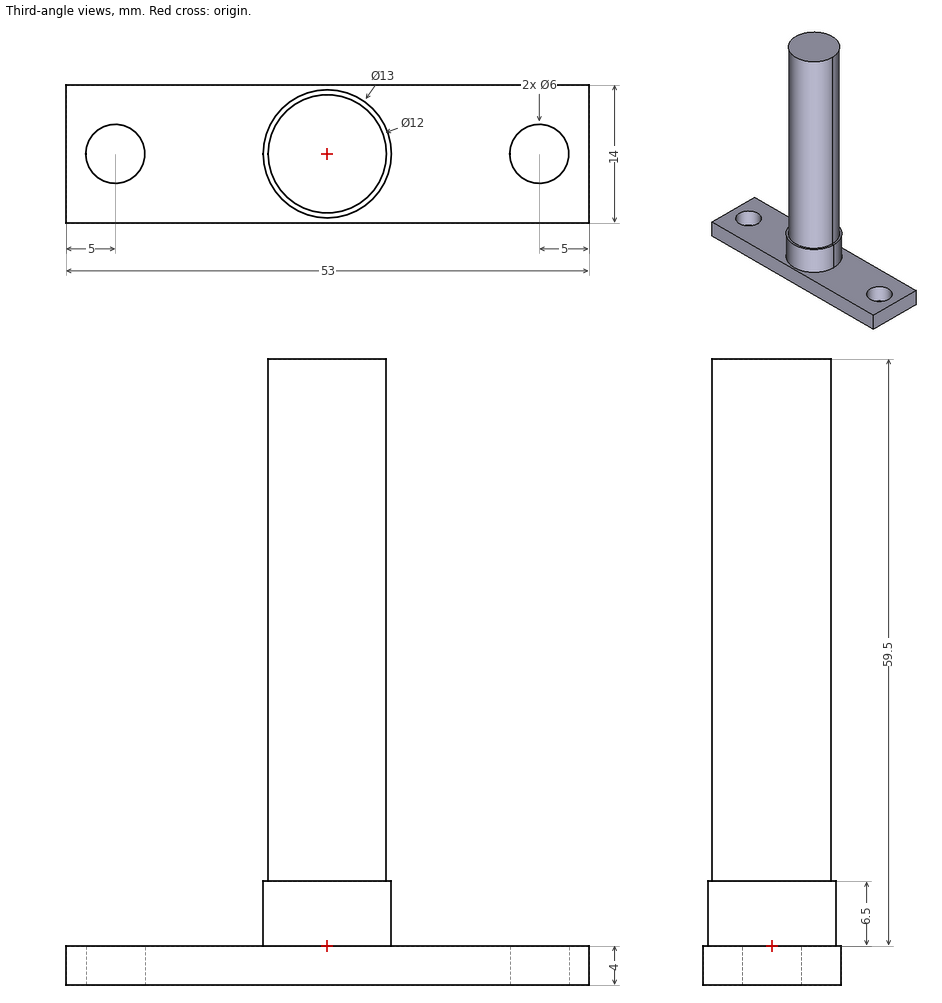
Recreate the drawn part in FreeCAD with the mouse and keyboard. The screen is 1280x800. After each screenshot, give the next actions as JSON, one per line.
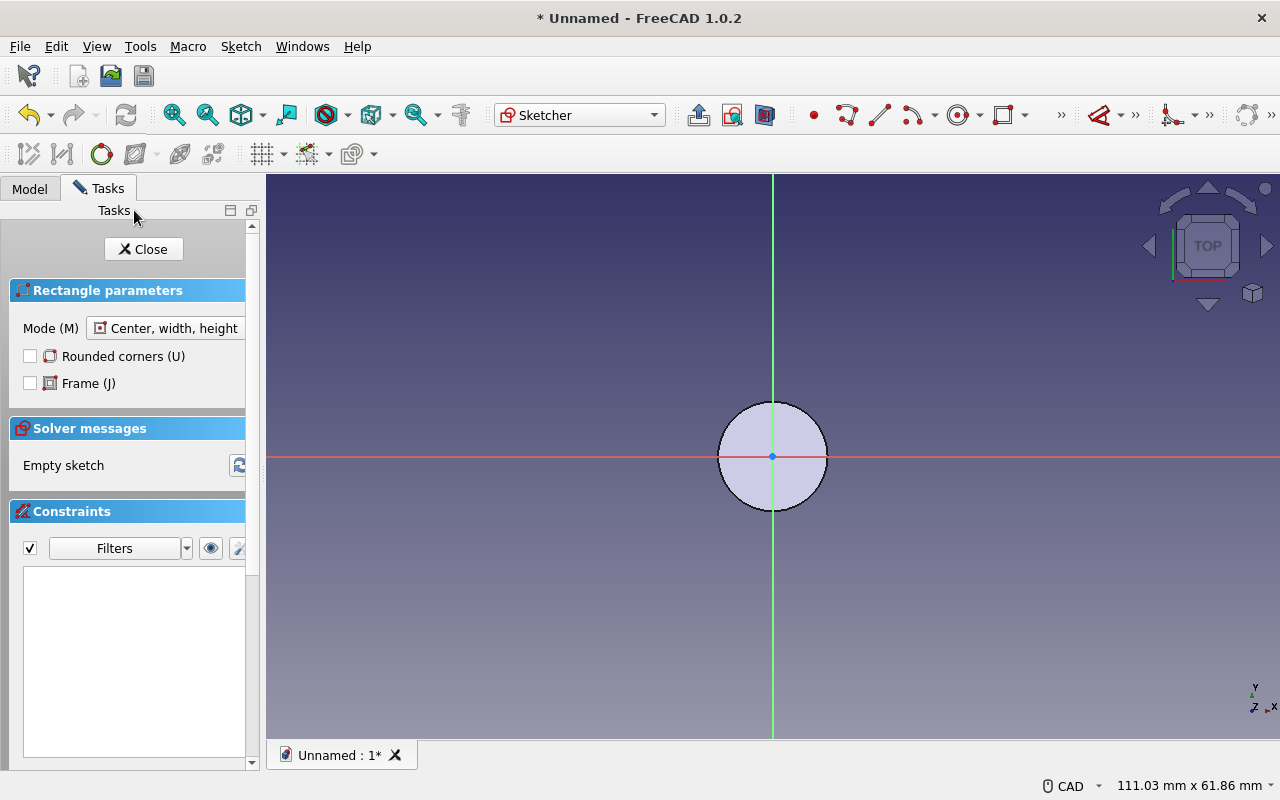
{"action": "left_click", "coordinate": [773, 456]}
{"action": "left_click", "coordinate": [1015, 393]}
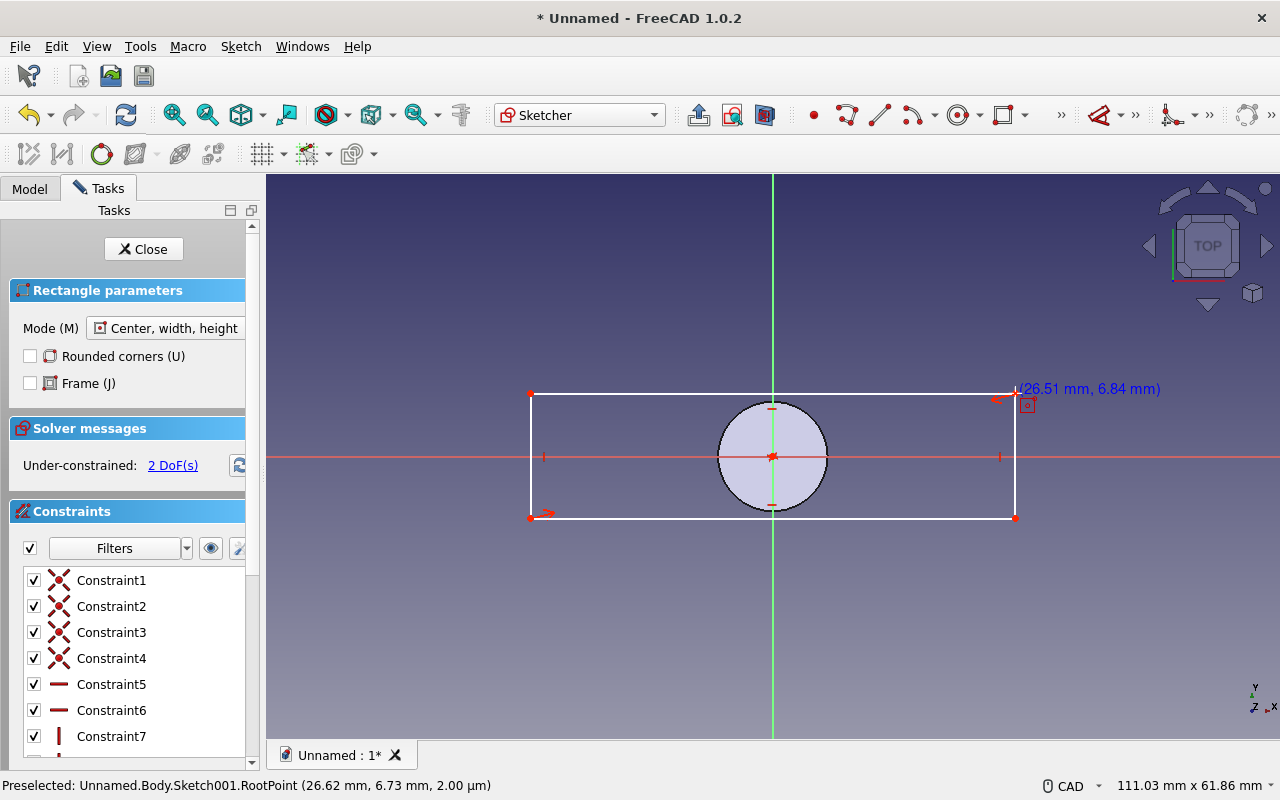
{"action": "key", "text": "g c"}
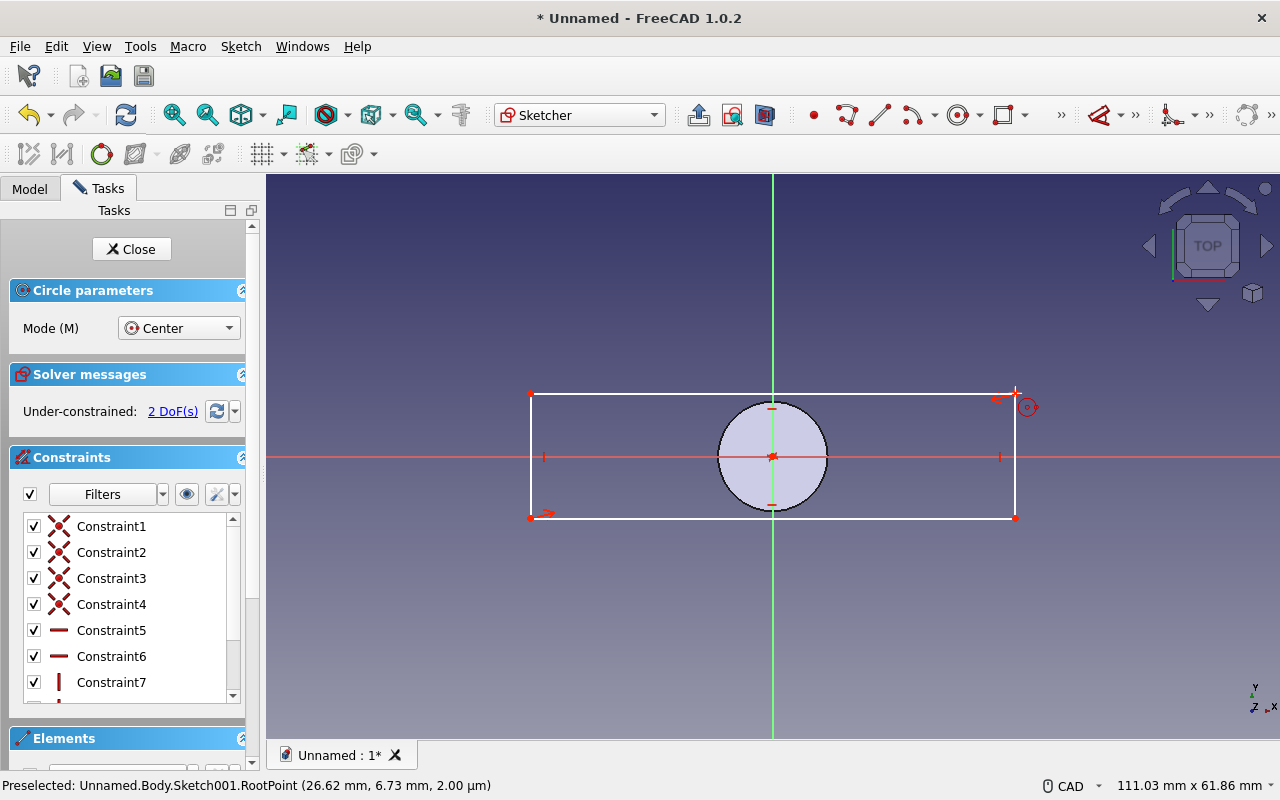
{"action": "left_click", "coordinate": [969, 456]}
{"action": "left_click", "coordinate": [989, 437]}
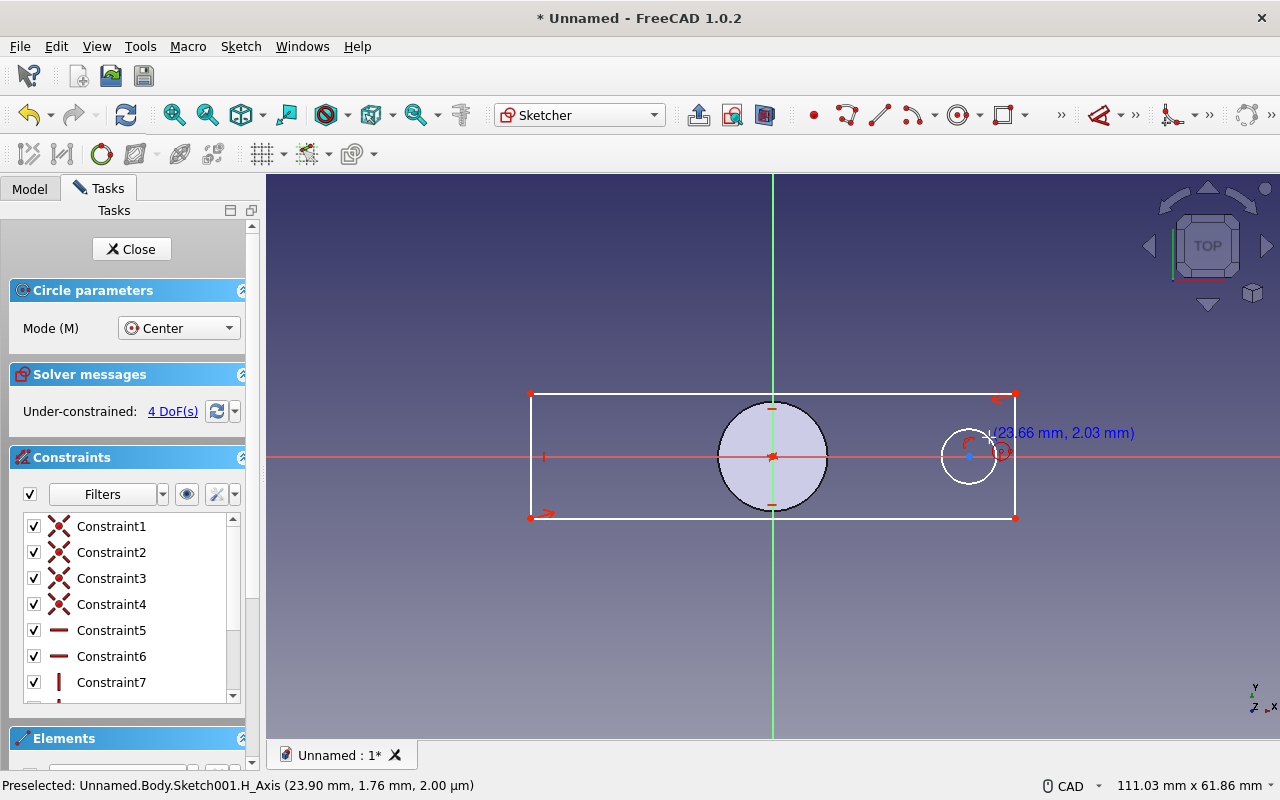
{"action": "left_click", "coordinate": [577, 456]}
{"action": "left_click", "coordinate": [596, 437]}
{"action": "key", "text": "Escape"}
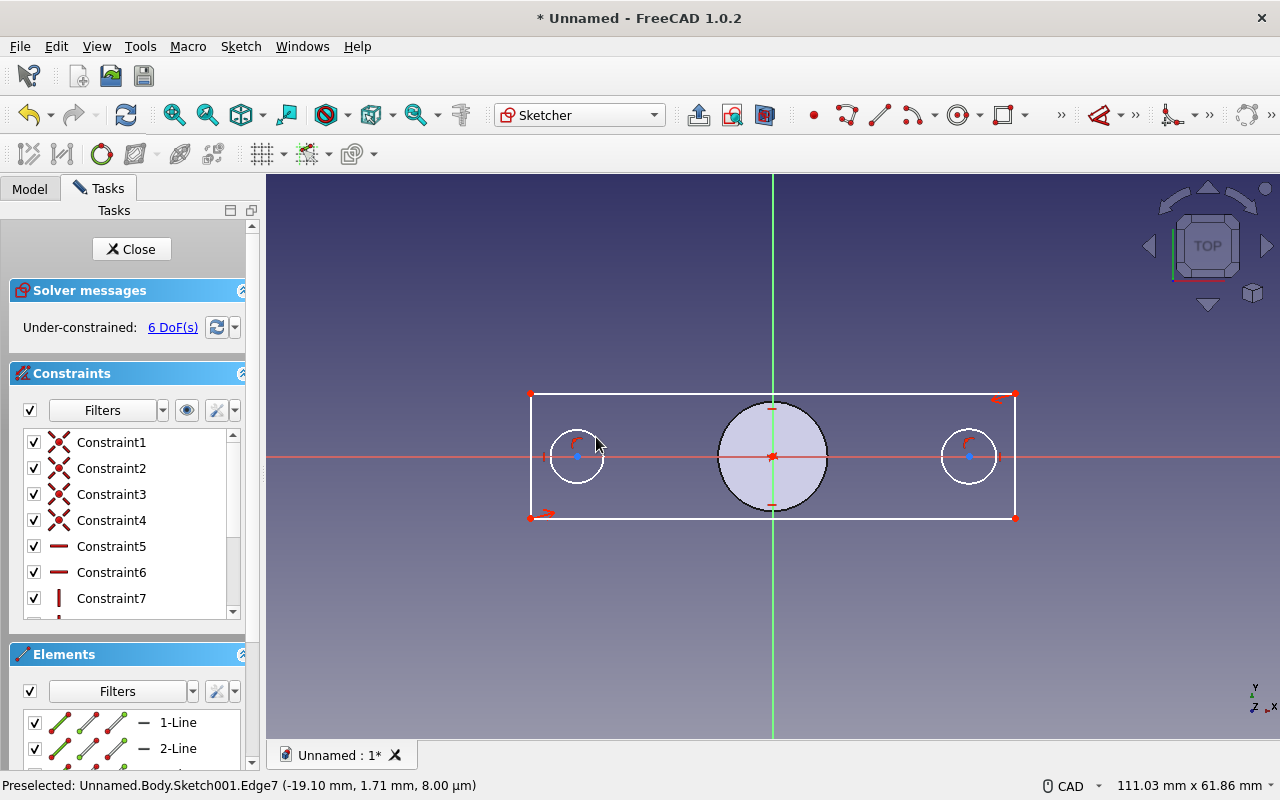
{"action": "left_click", "coordinate": [988, 437]}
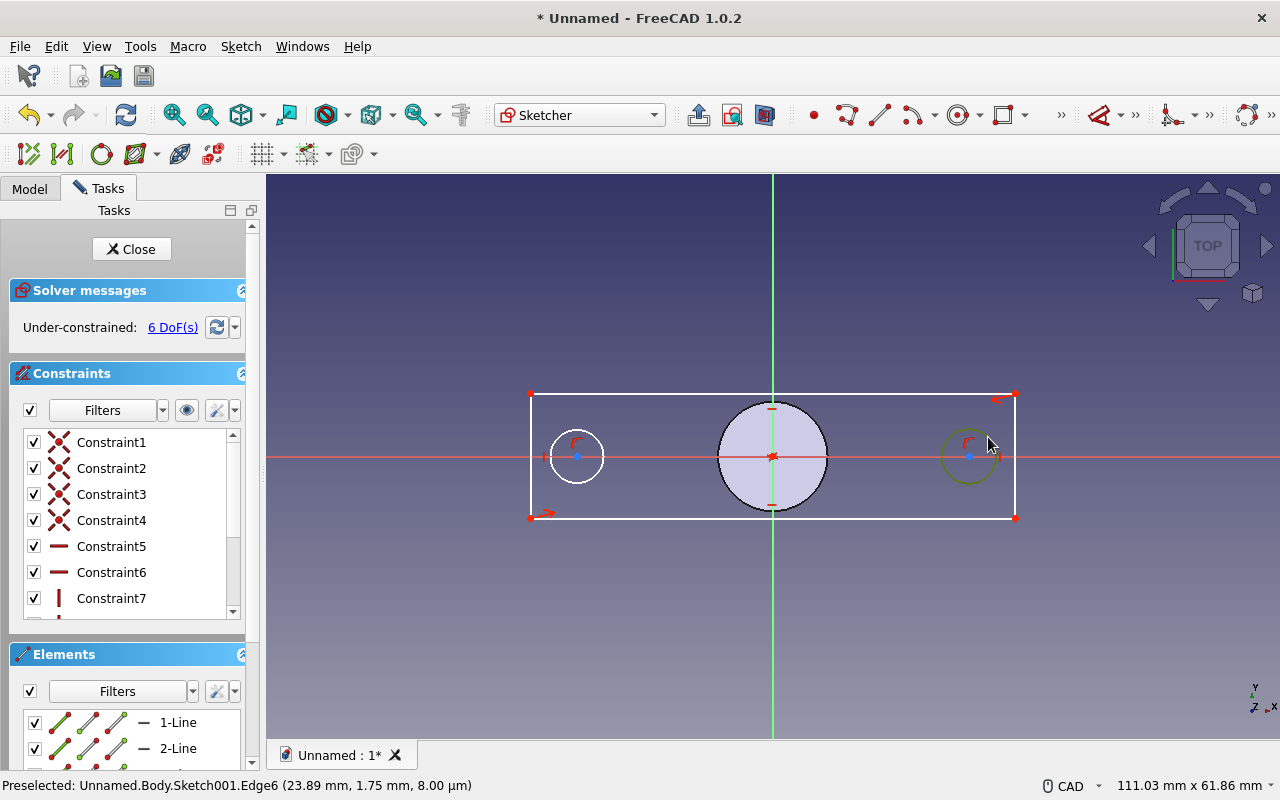
{"action": "left_click", "coordinate": [596, 438]}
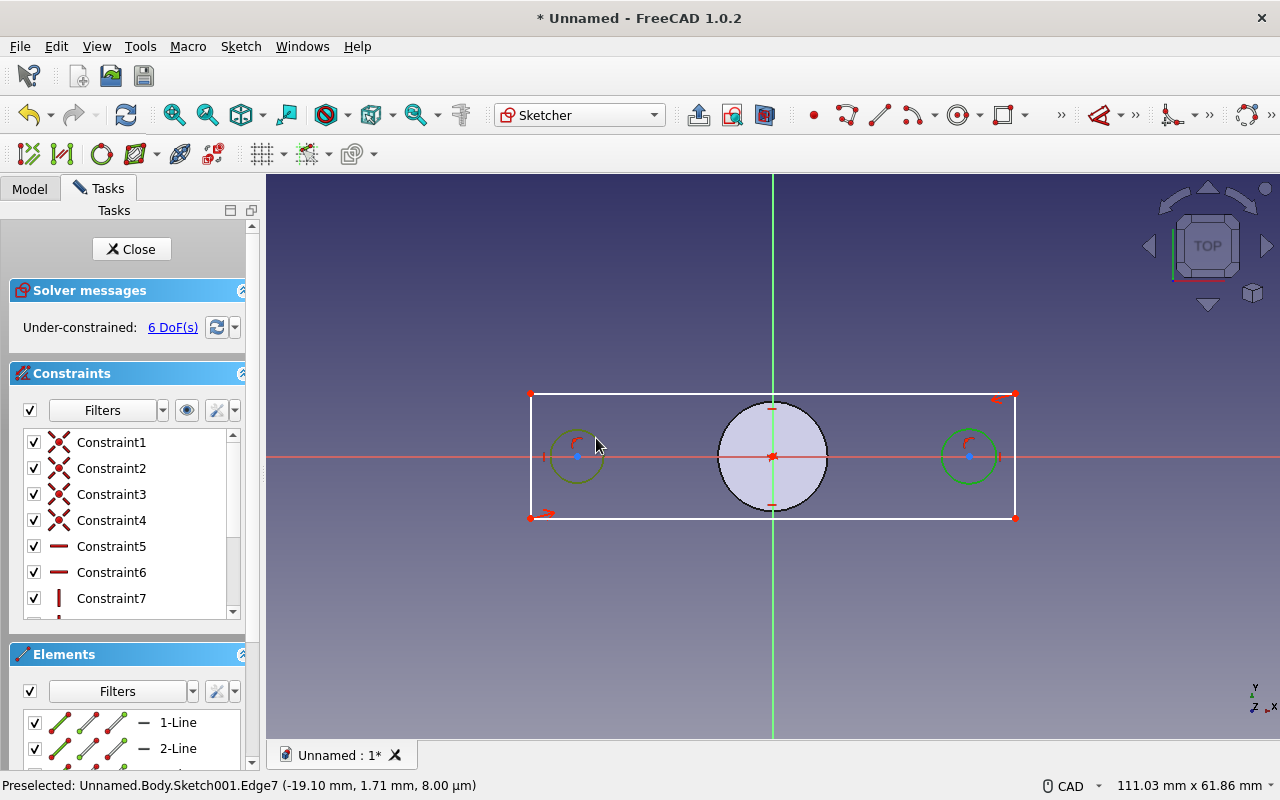
{"action": "key", "text": "e"}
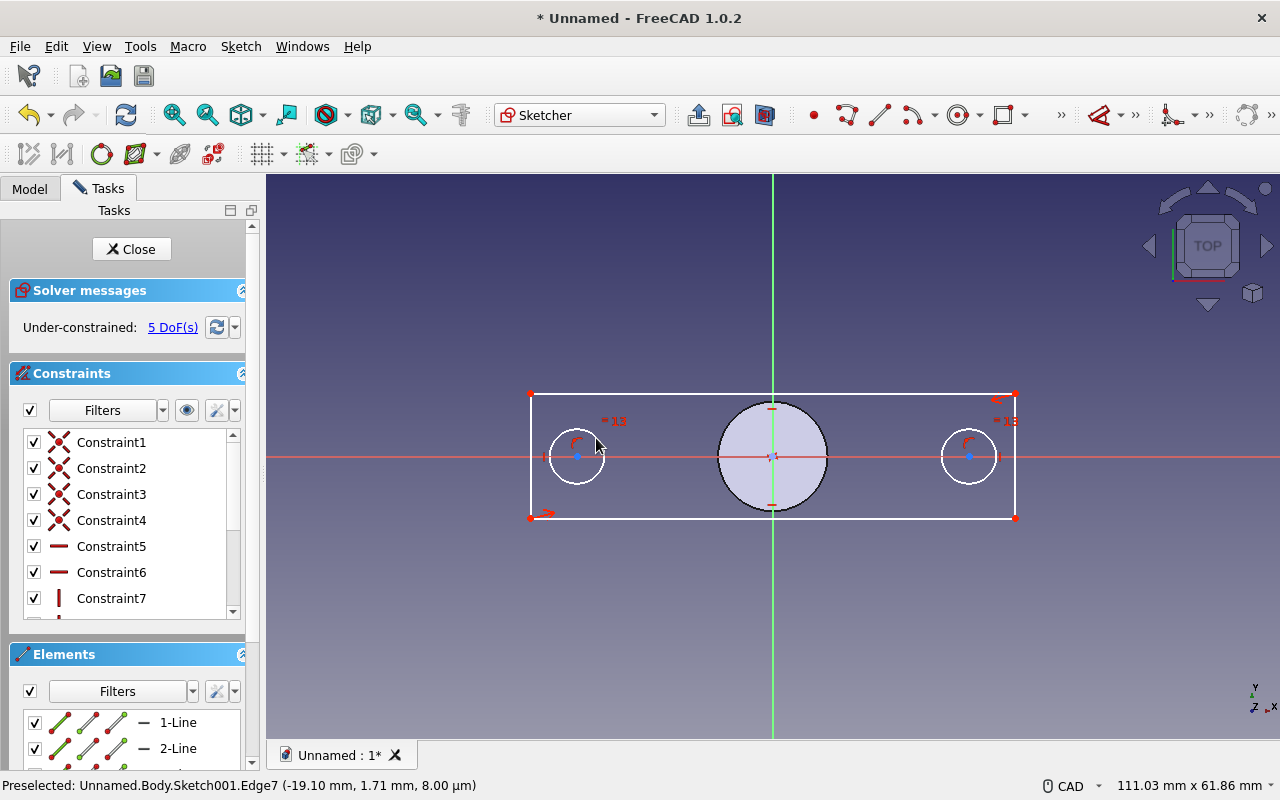
{"action": "key", "text": "d"}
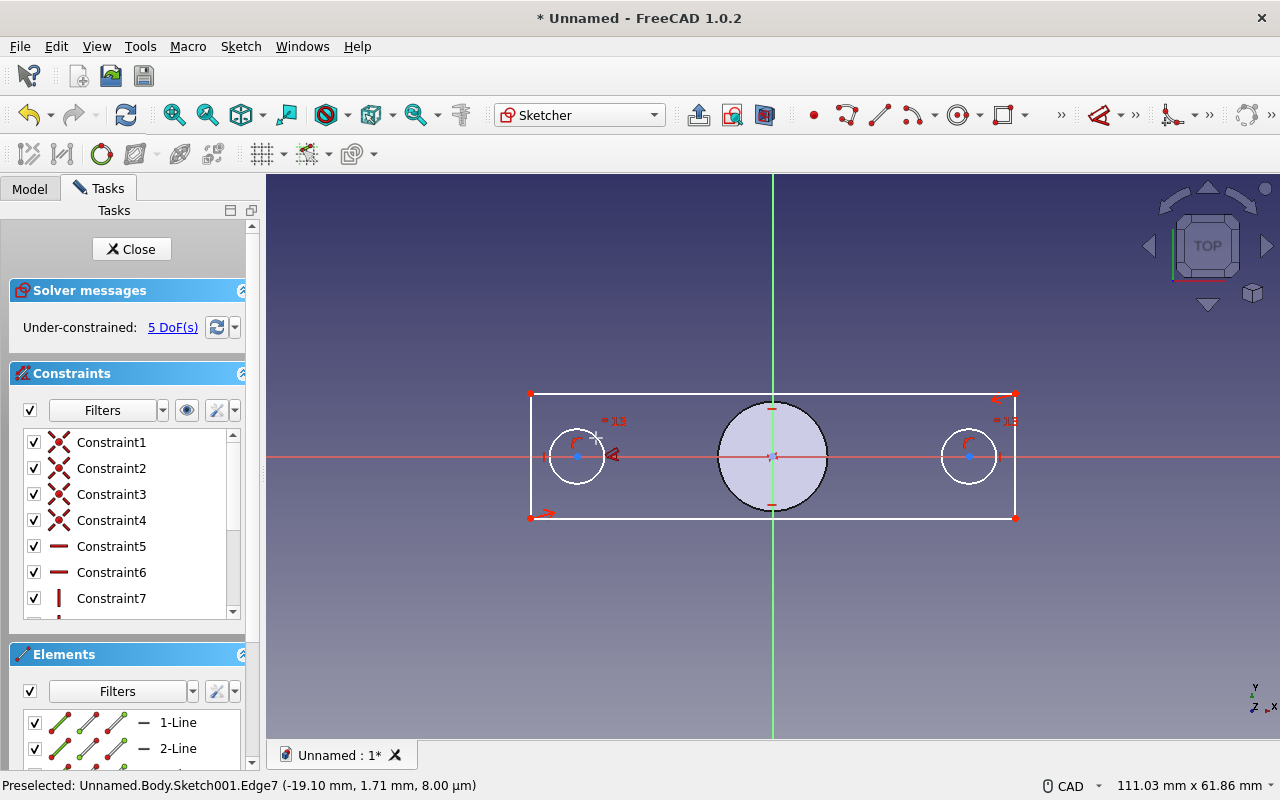
{"action": "left_click", "coordinate": [988, 437]}
{"action": "left_click", "coordinate": [927, 415]}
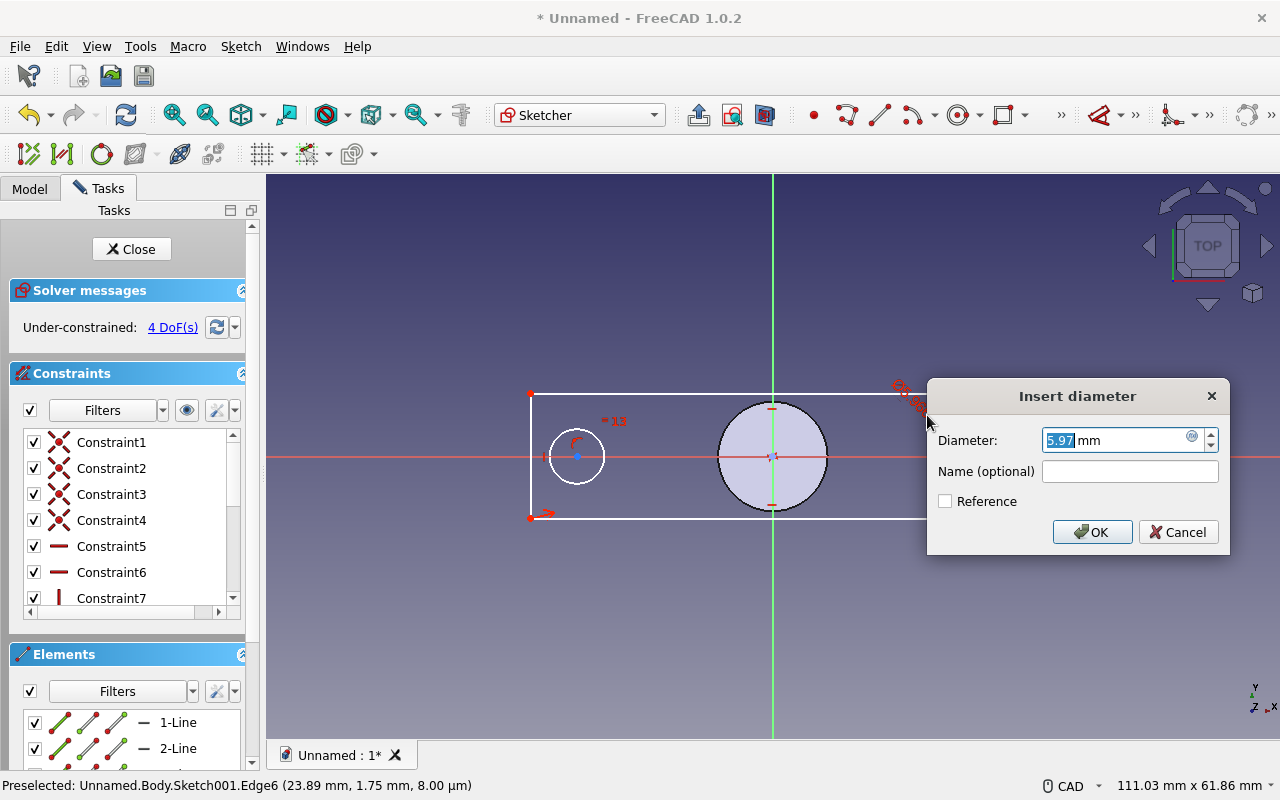
{"action": "type", "text": "6"}
{"action": "key", "text": "Return"}